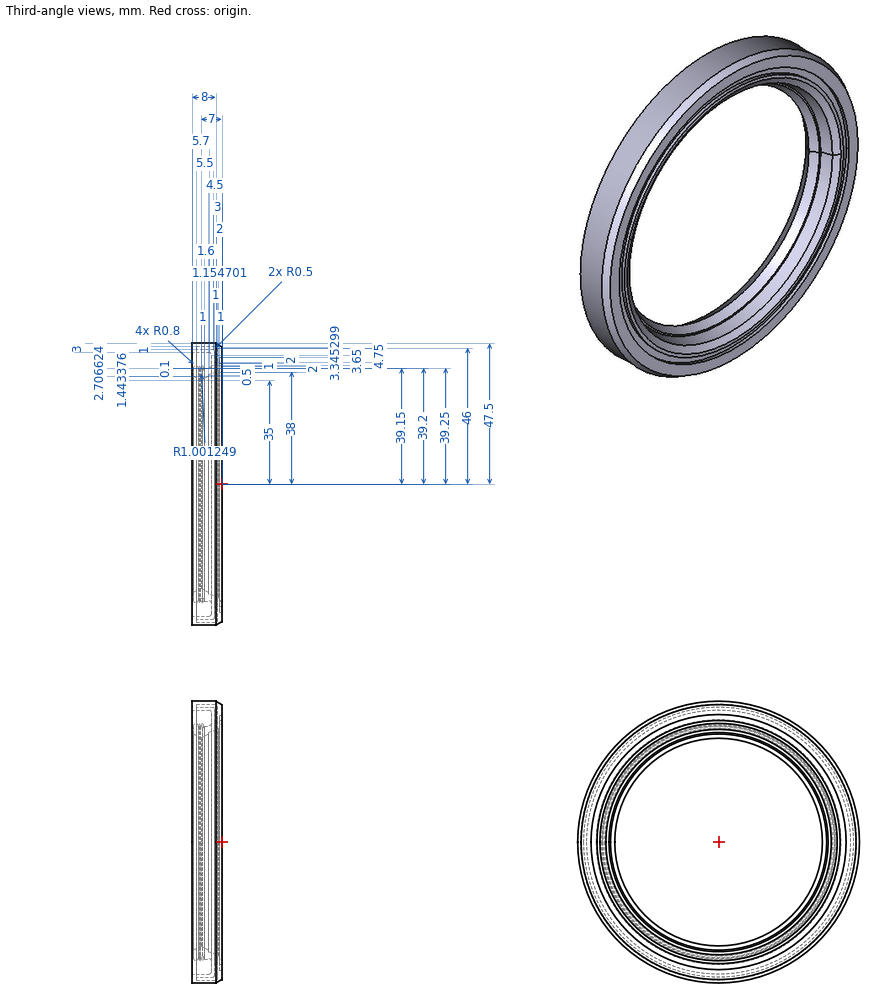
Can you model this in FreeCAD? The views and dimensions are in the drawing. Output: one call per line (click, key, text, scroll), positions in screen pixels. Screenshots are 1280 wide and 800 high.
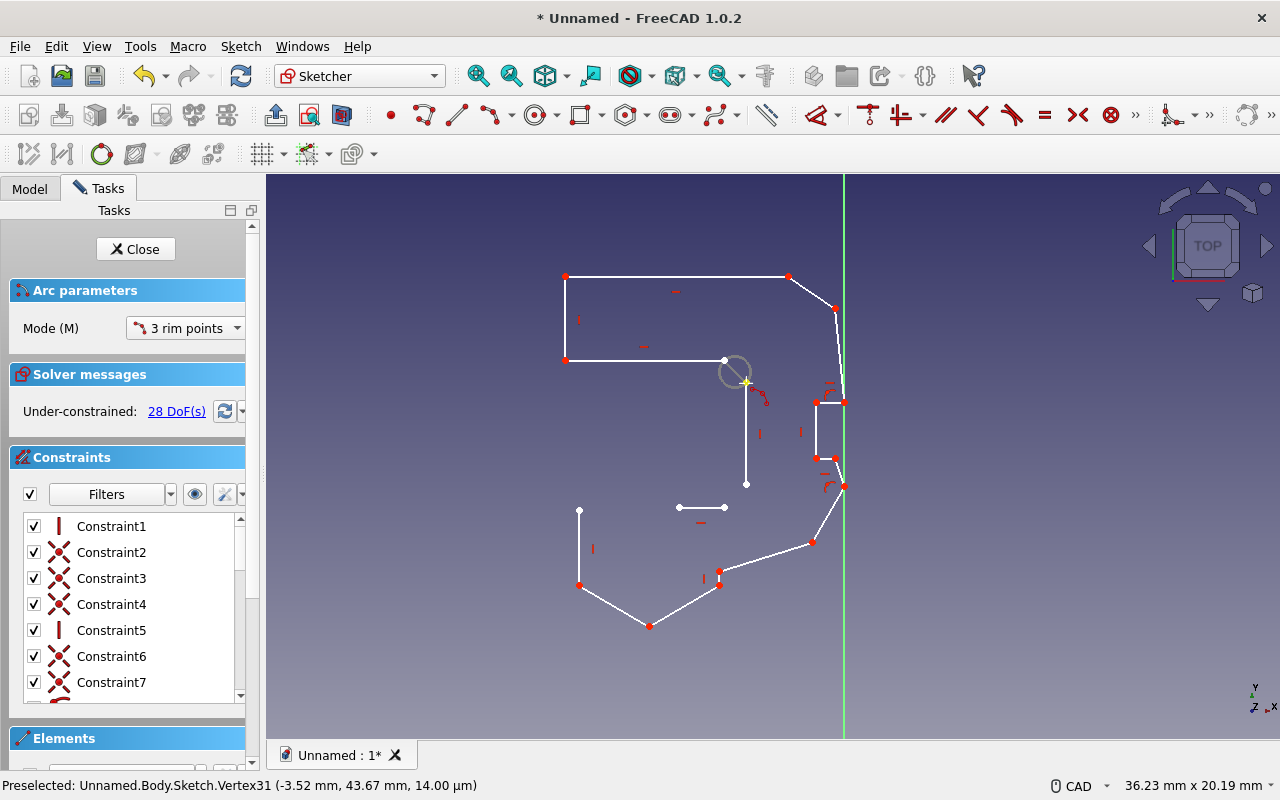
scroll(740, 366, up, 5)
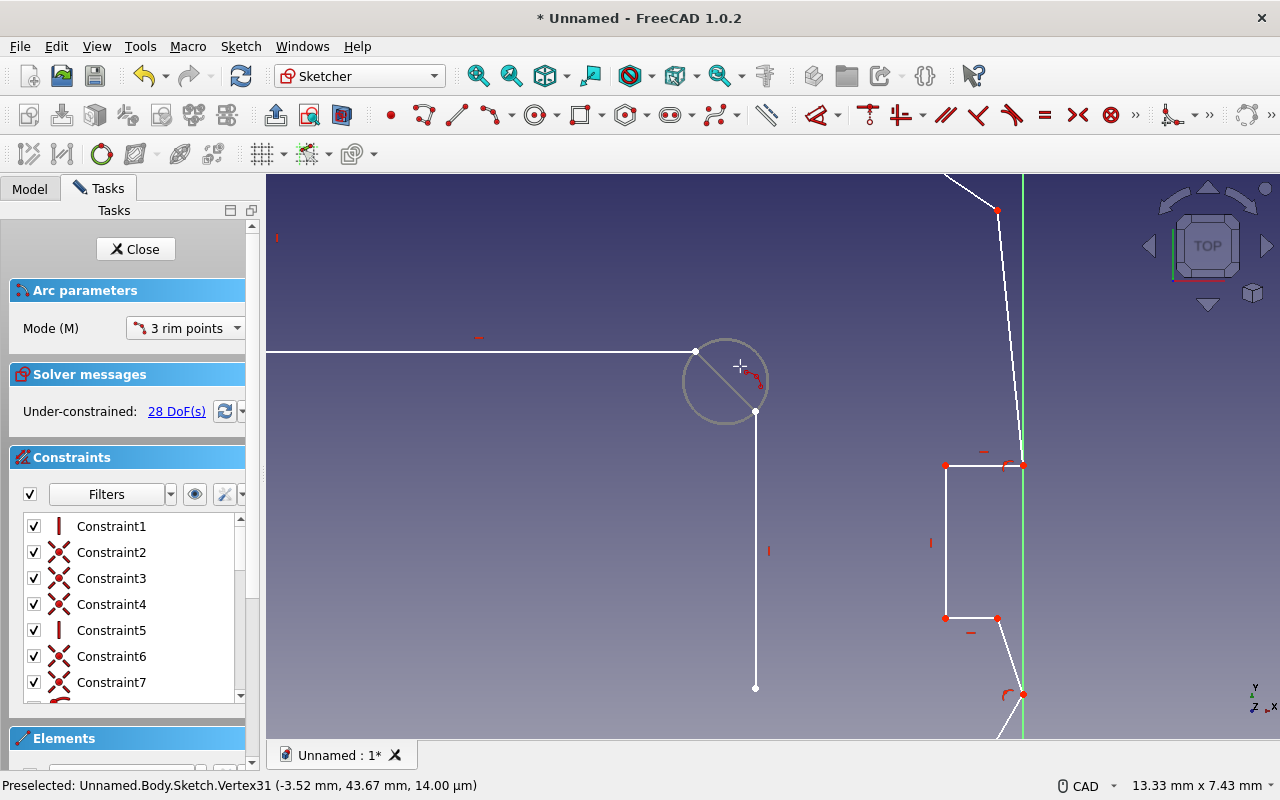
click(739, 367)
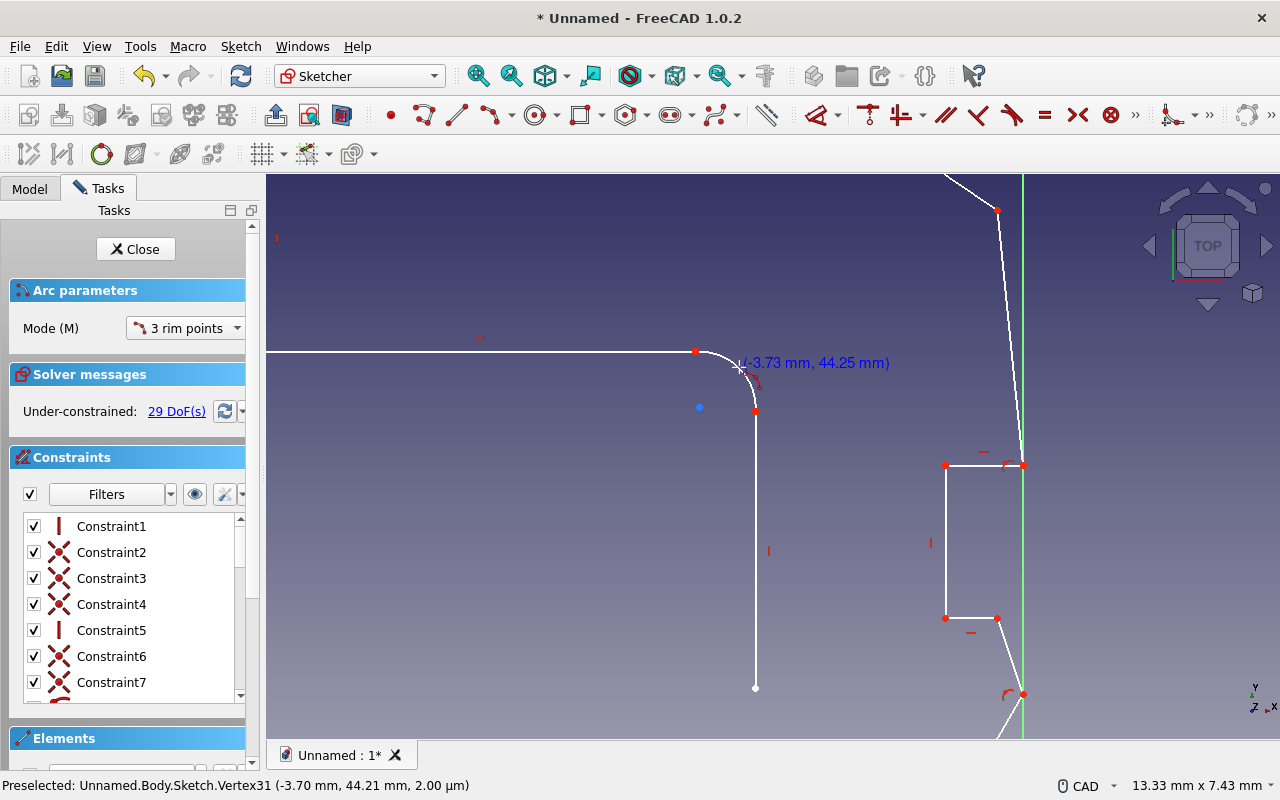
click(756, 689)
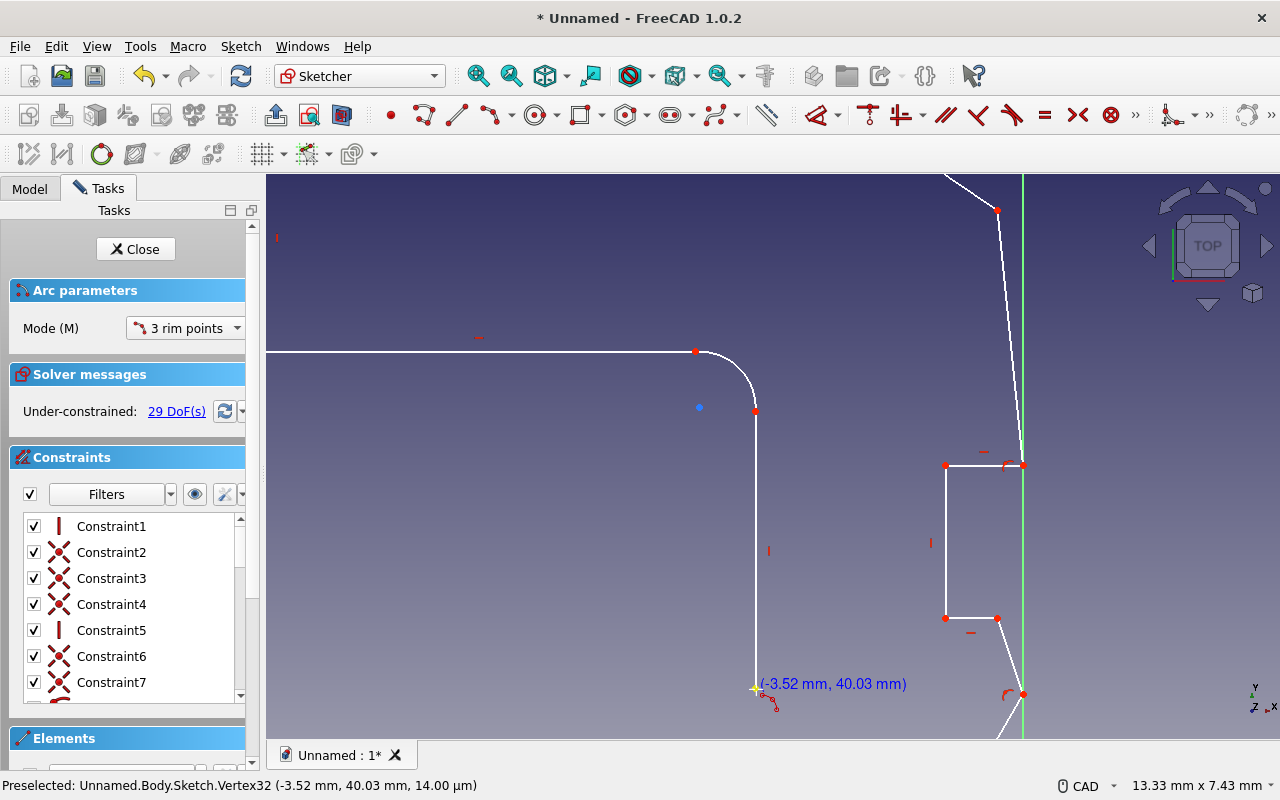
scroll(740, 375, down, 5)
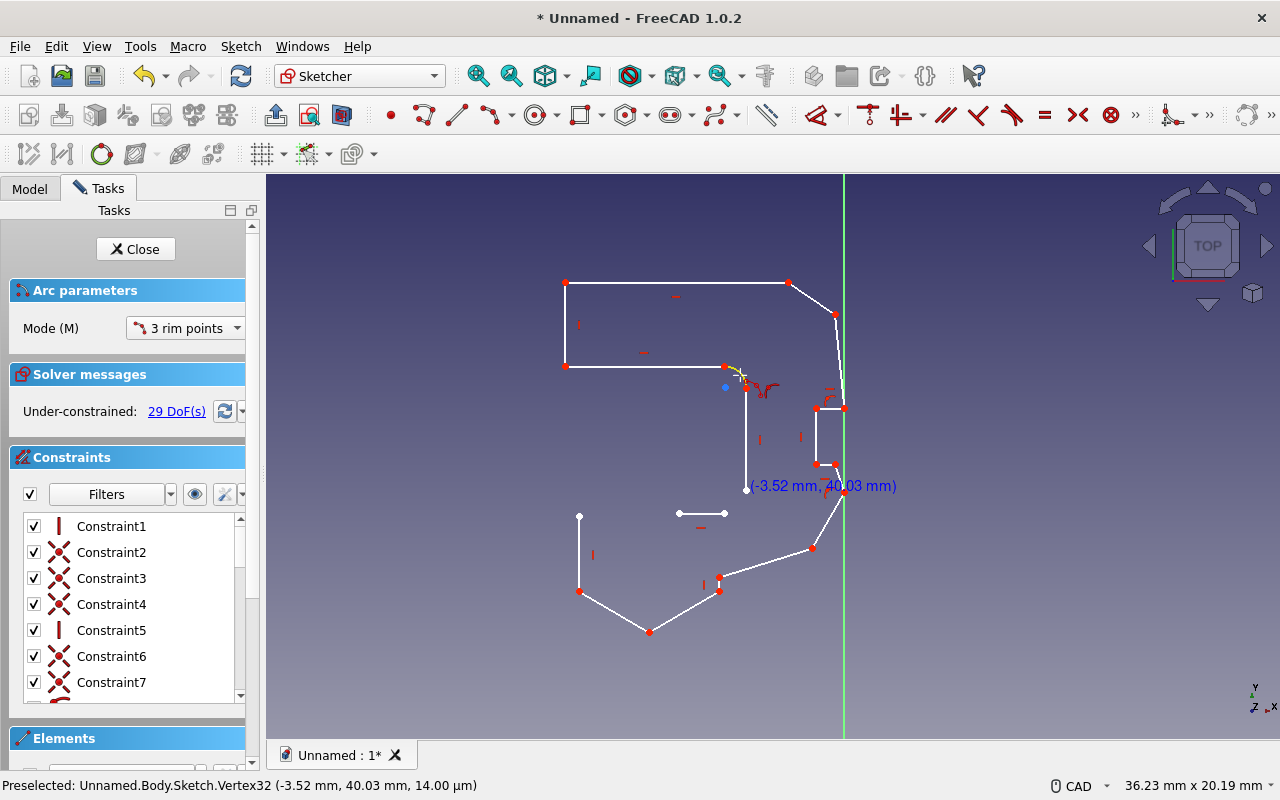
click(724, 514)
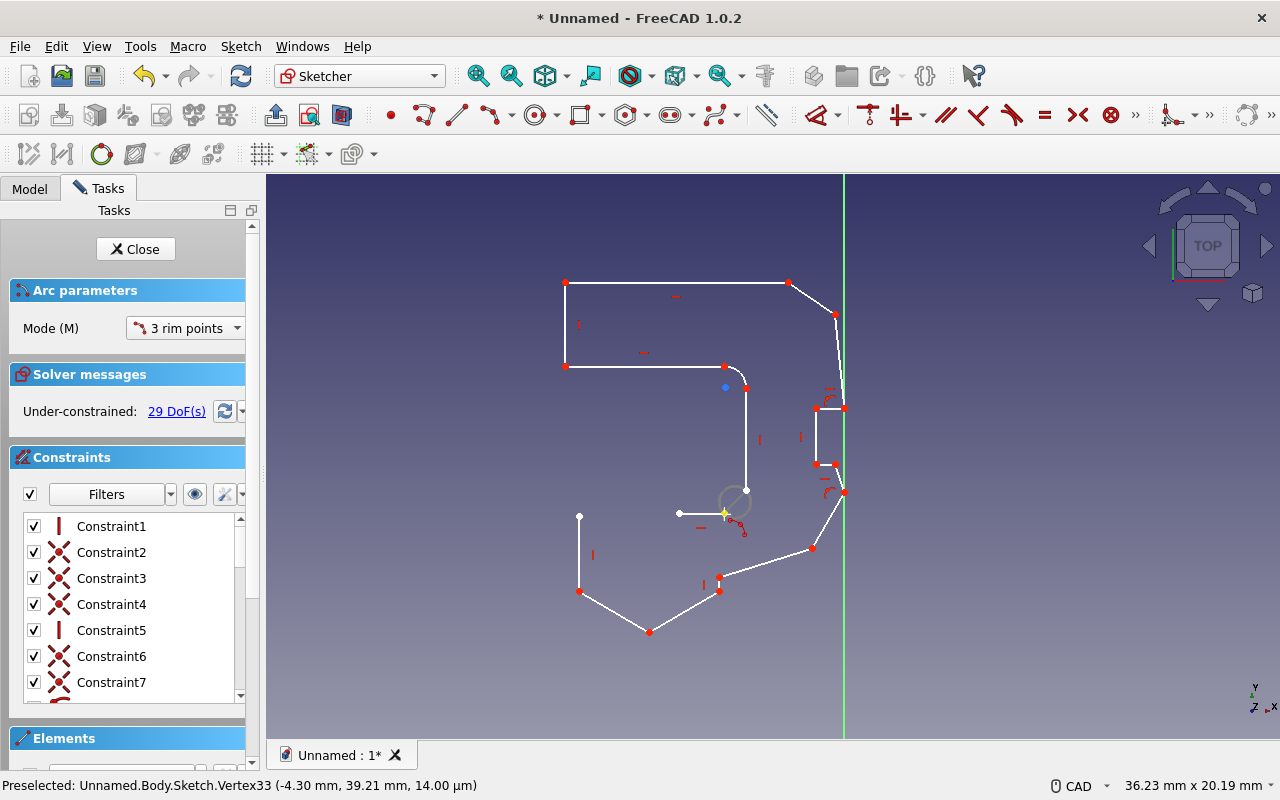
scroll(740, 506, up, 5)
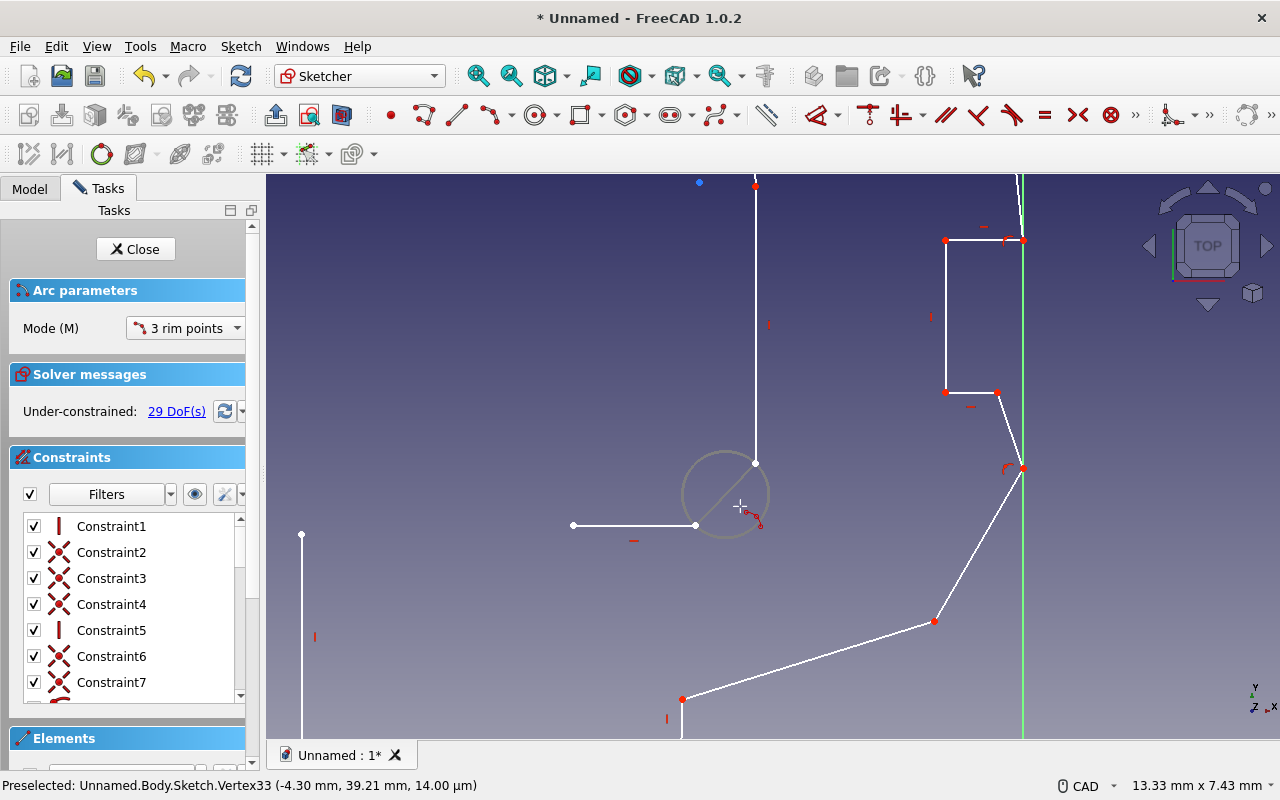
click(739, 505)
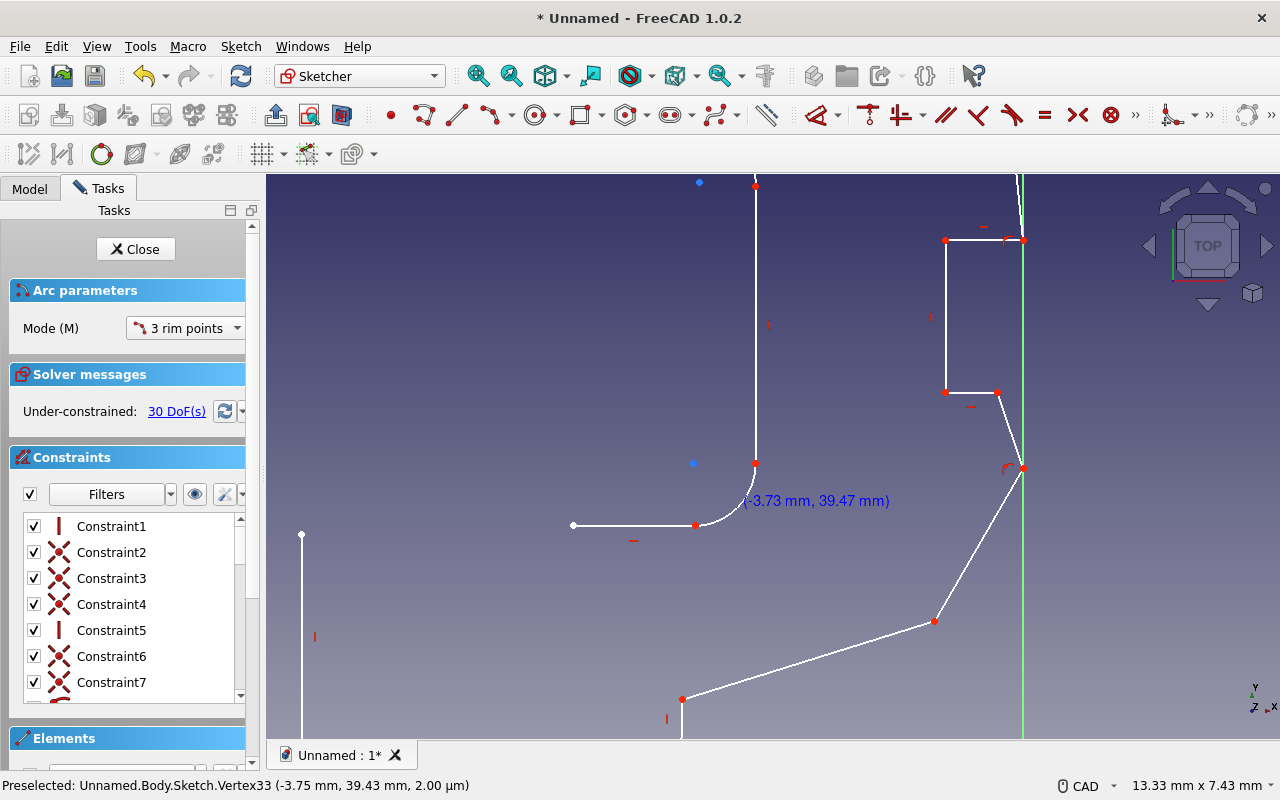
click(573, 526)
click(422, 530)
click(502, 603)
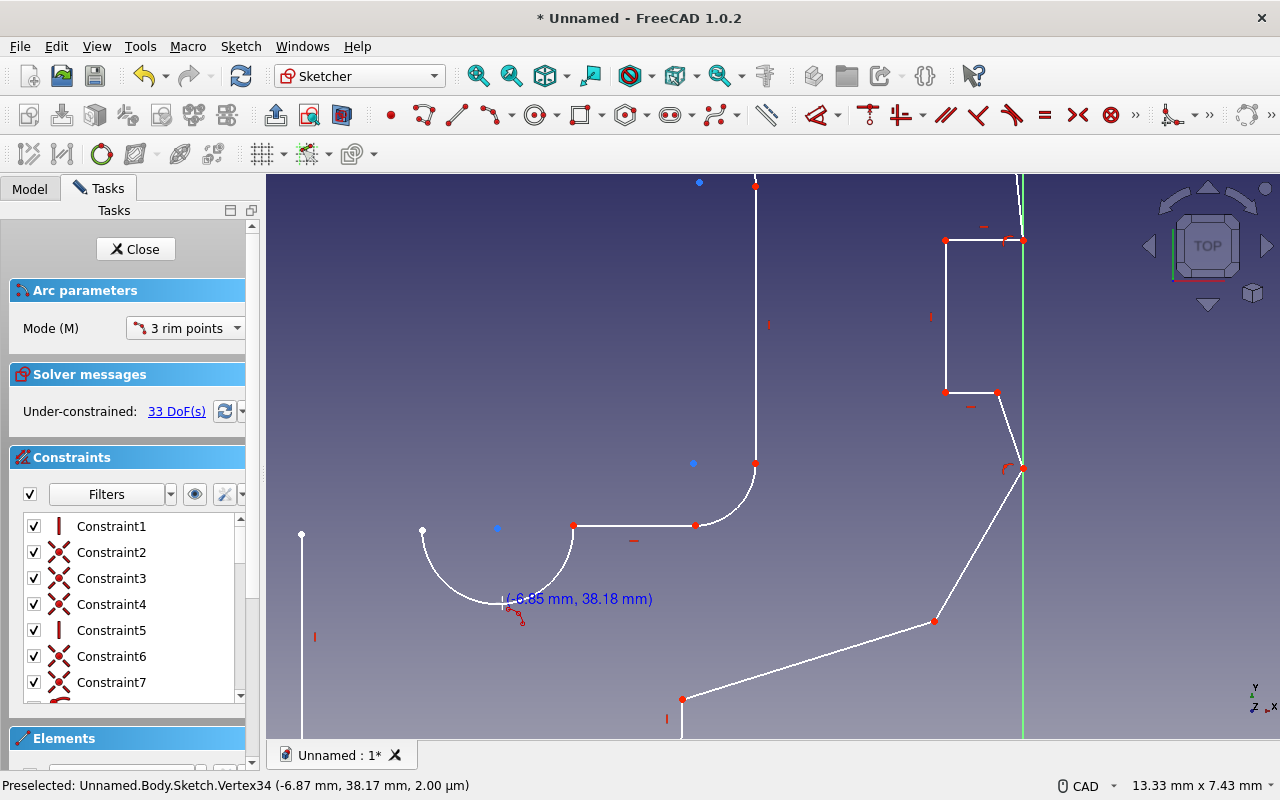
click(422, 531)
click(302, 534)
click(361, 469)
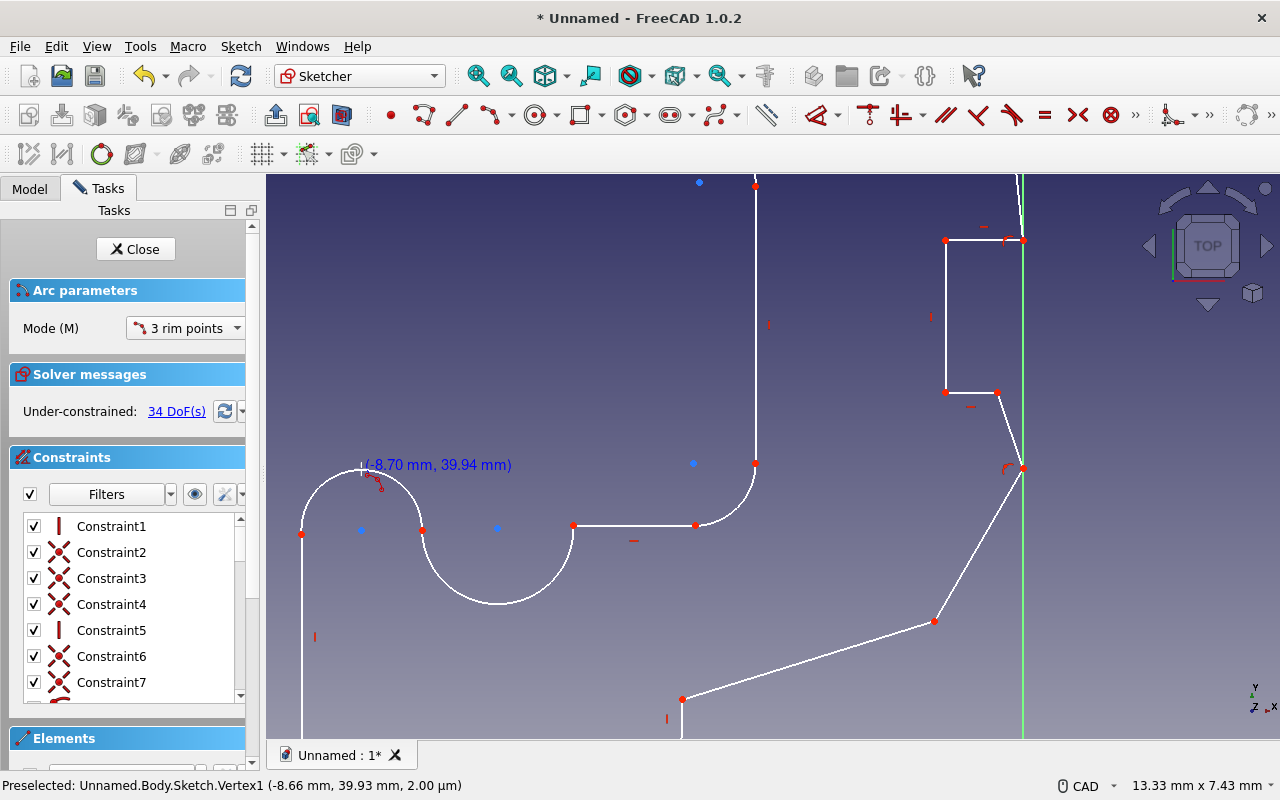
click(424, 116)